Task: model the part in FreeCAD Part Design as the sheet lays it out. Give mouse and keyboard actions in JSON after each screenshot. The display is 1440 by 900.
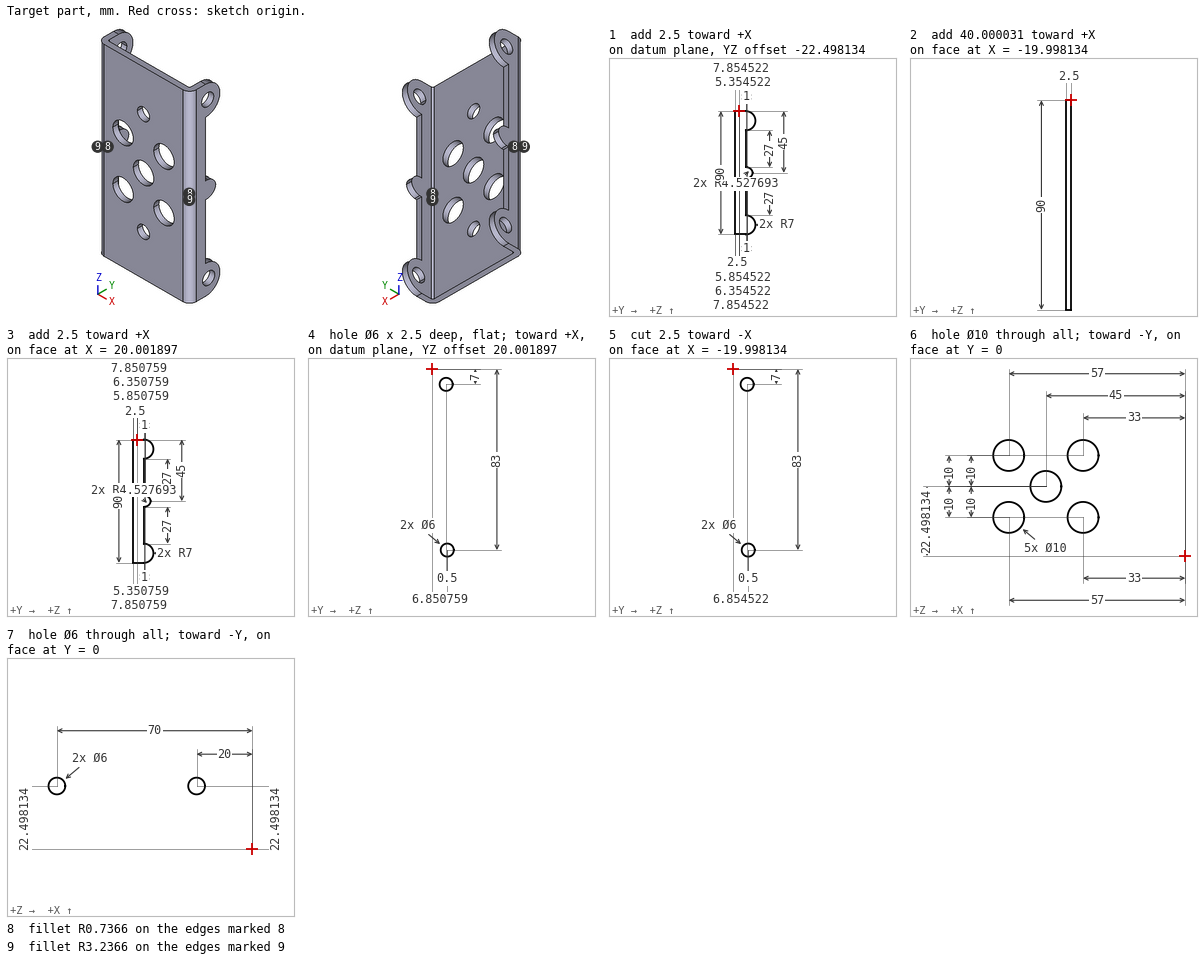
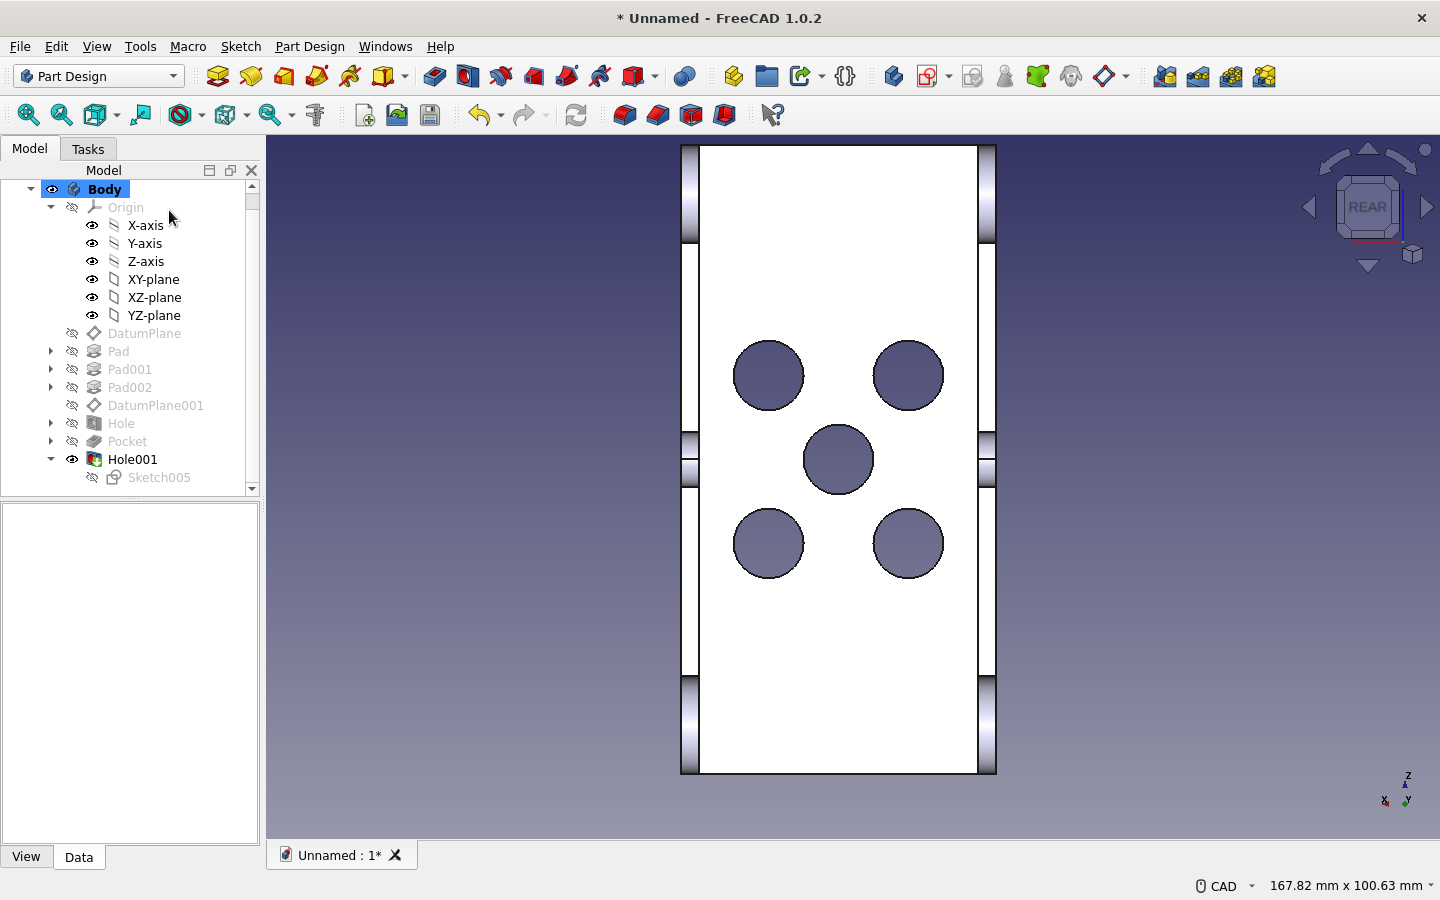
{"action": "left_click", "coordinate": [838, 279]}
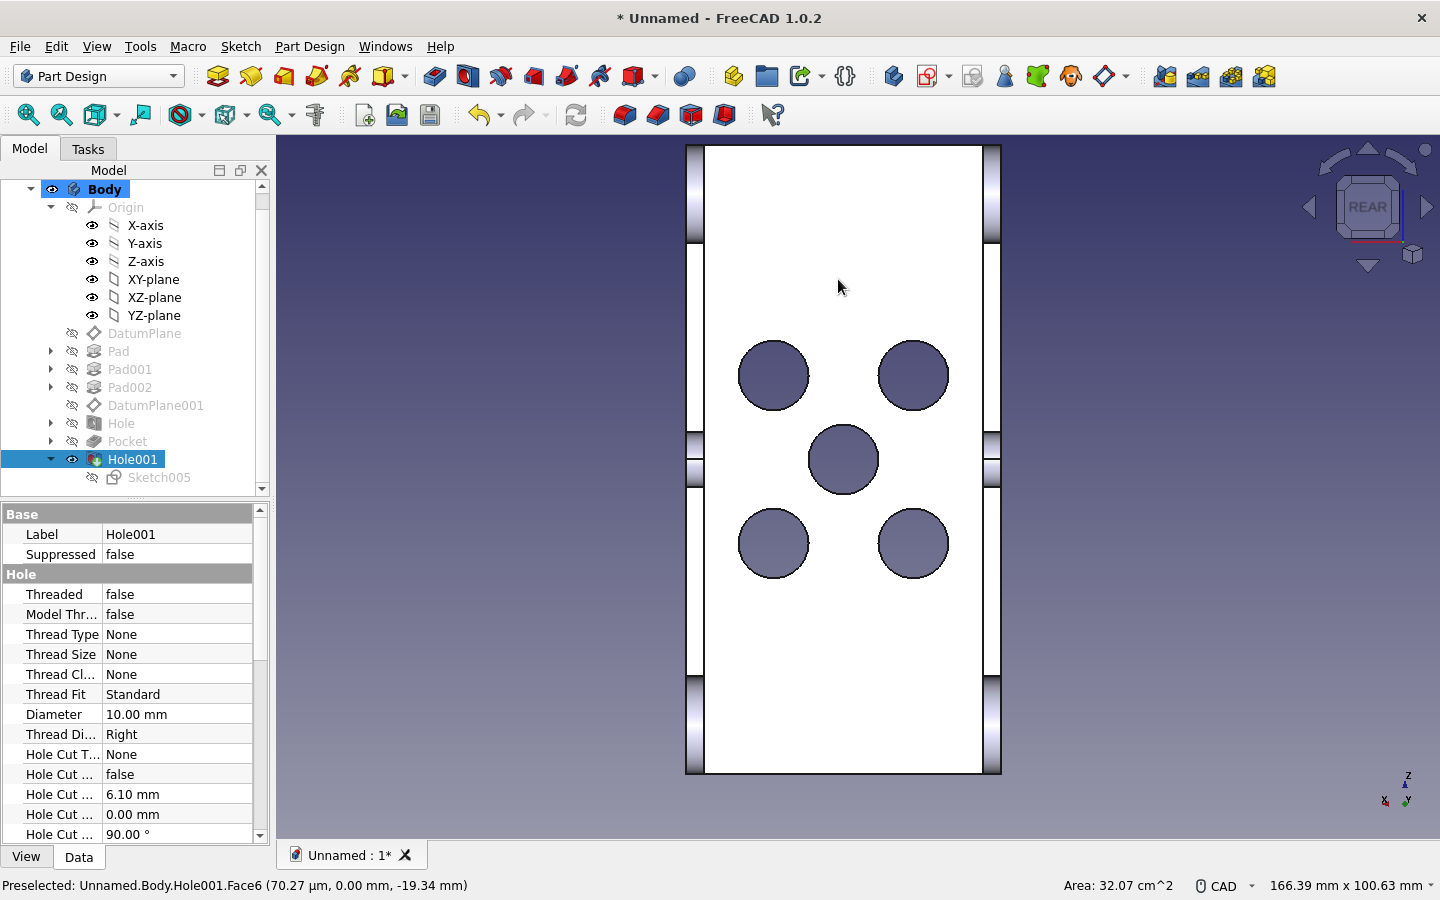
{"action": "left_click", "coordinate": [926, 76]}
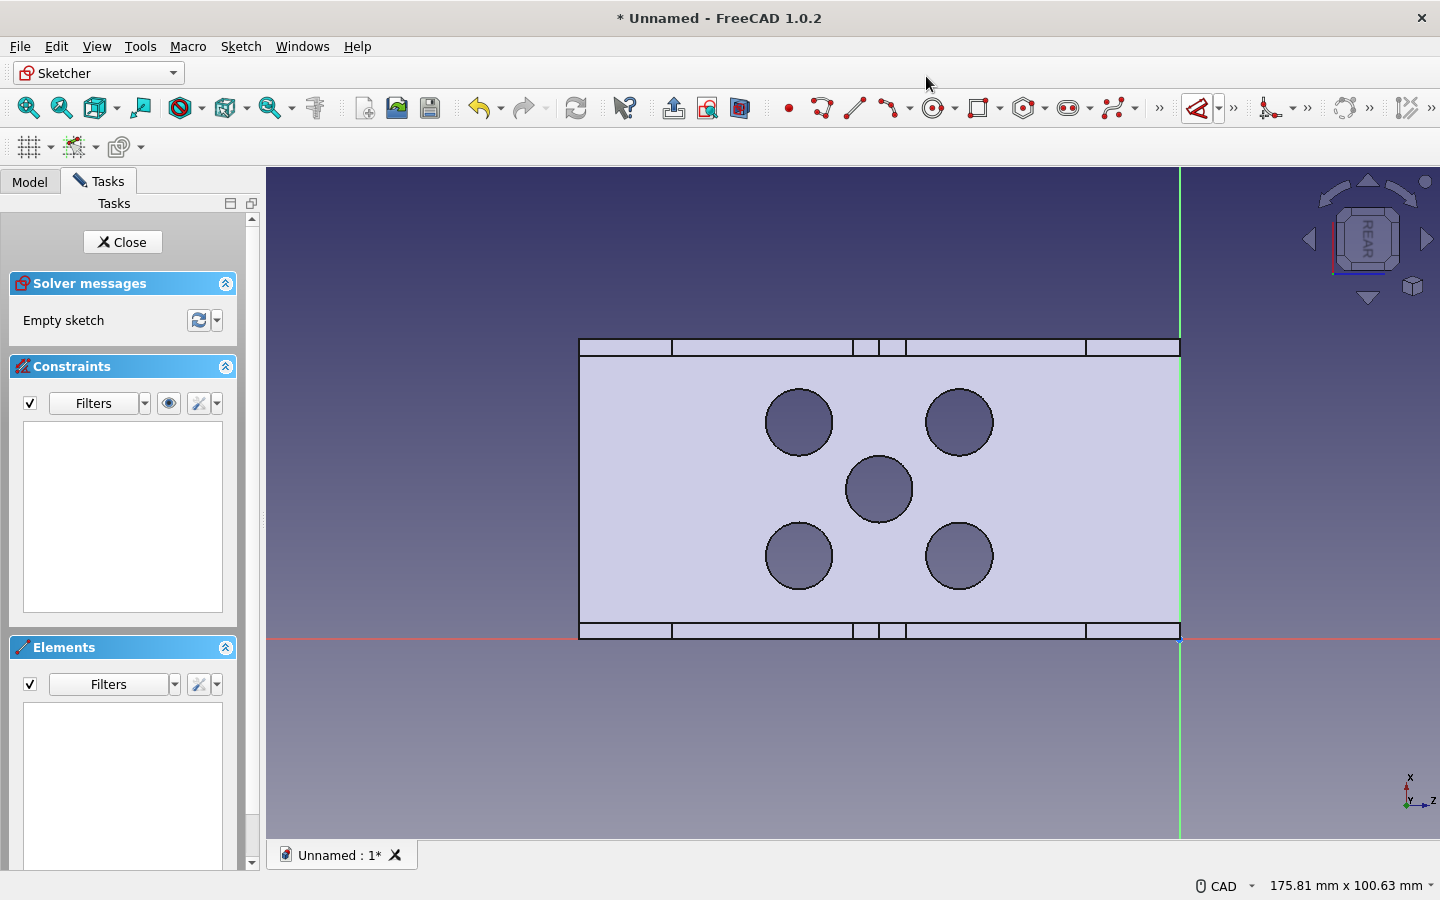
{"action": "scroll", "coordinate": [1244, 658], "scroll_direction": "up", "scroll_amount": 2}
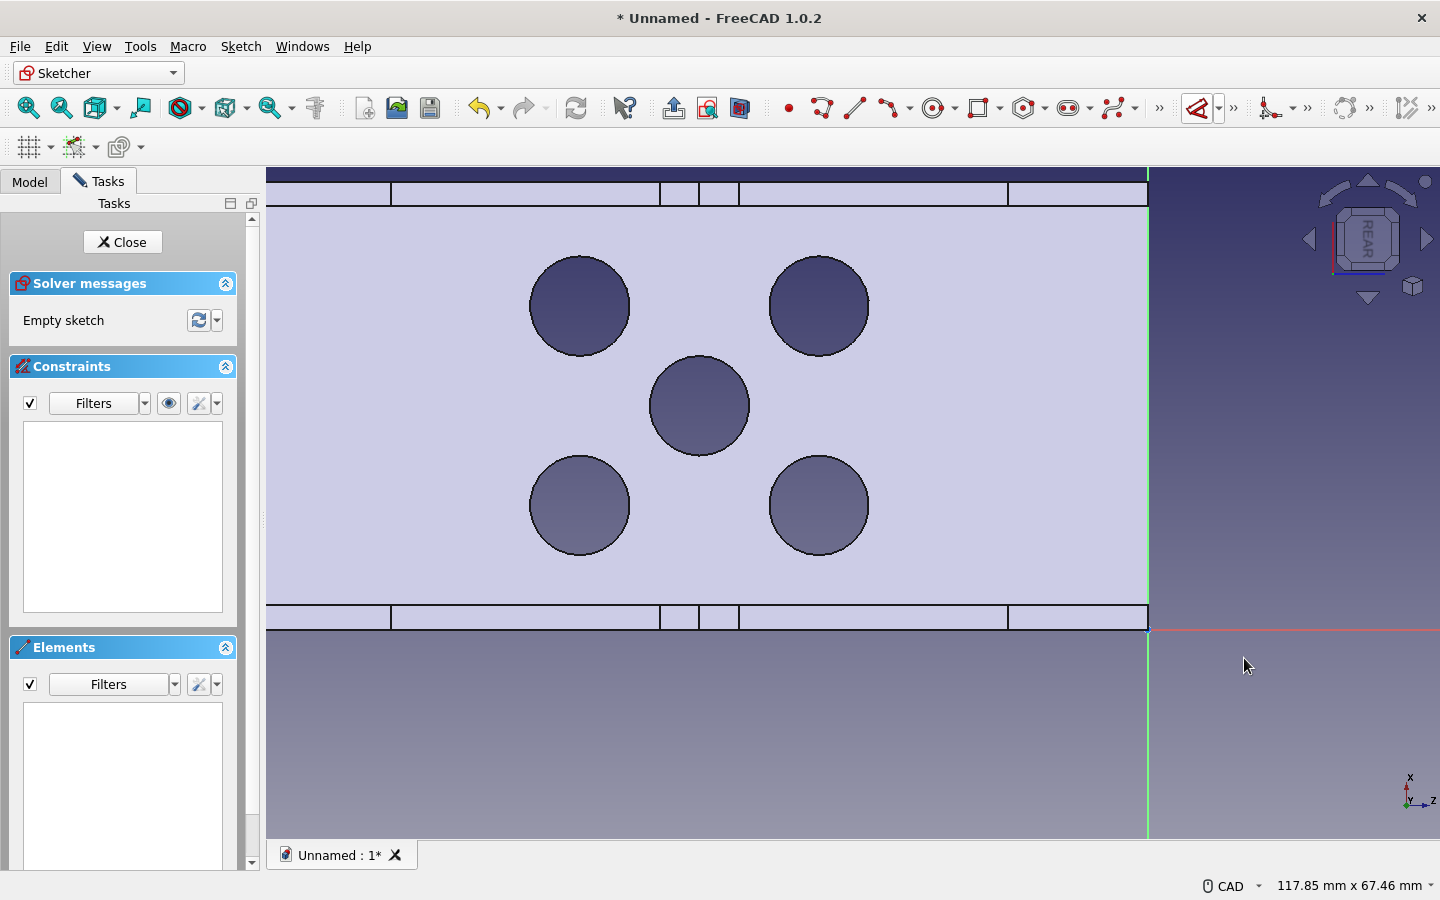
{"action": "left_click", "coordinate": [932, 108]}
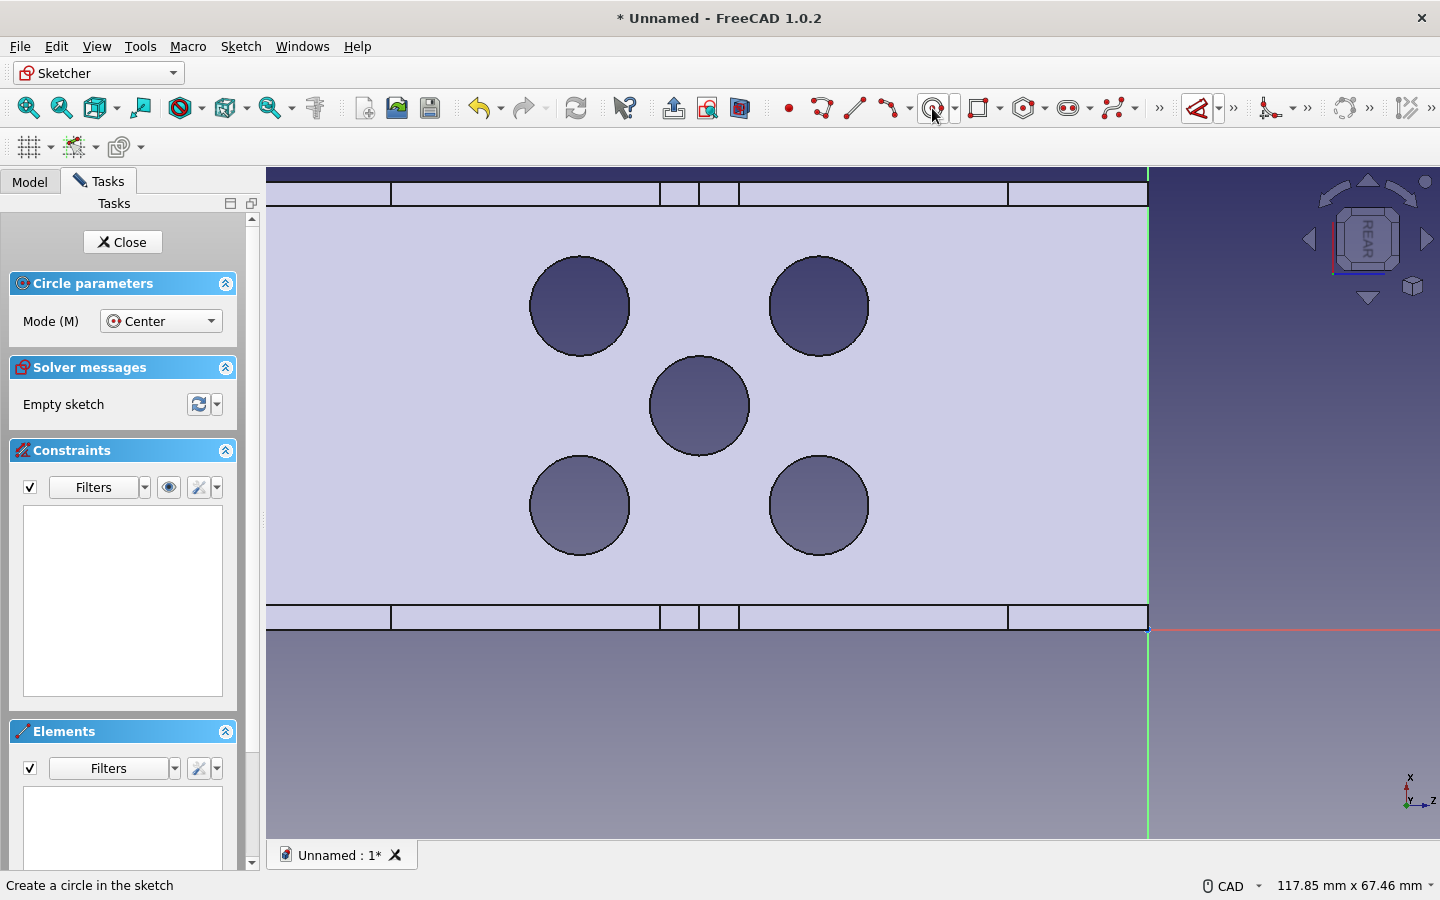
{"action": "left_click", "coordinate": [450, 406]}
{"action": "mouse_move", "coordinate": [472, 385]}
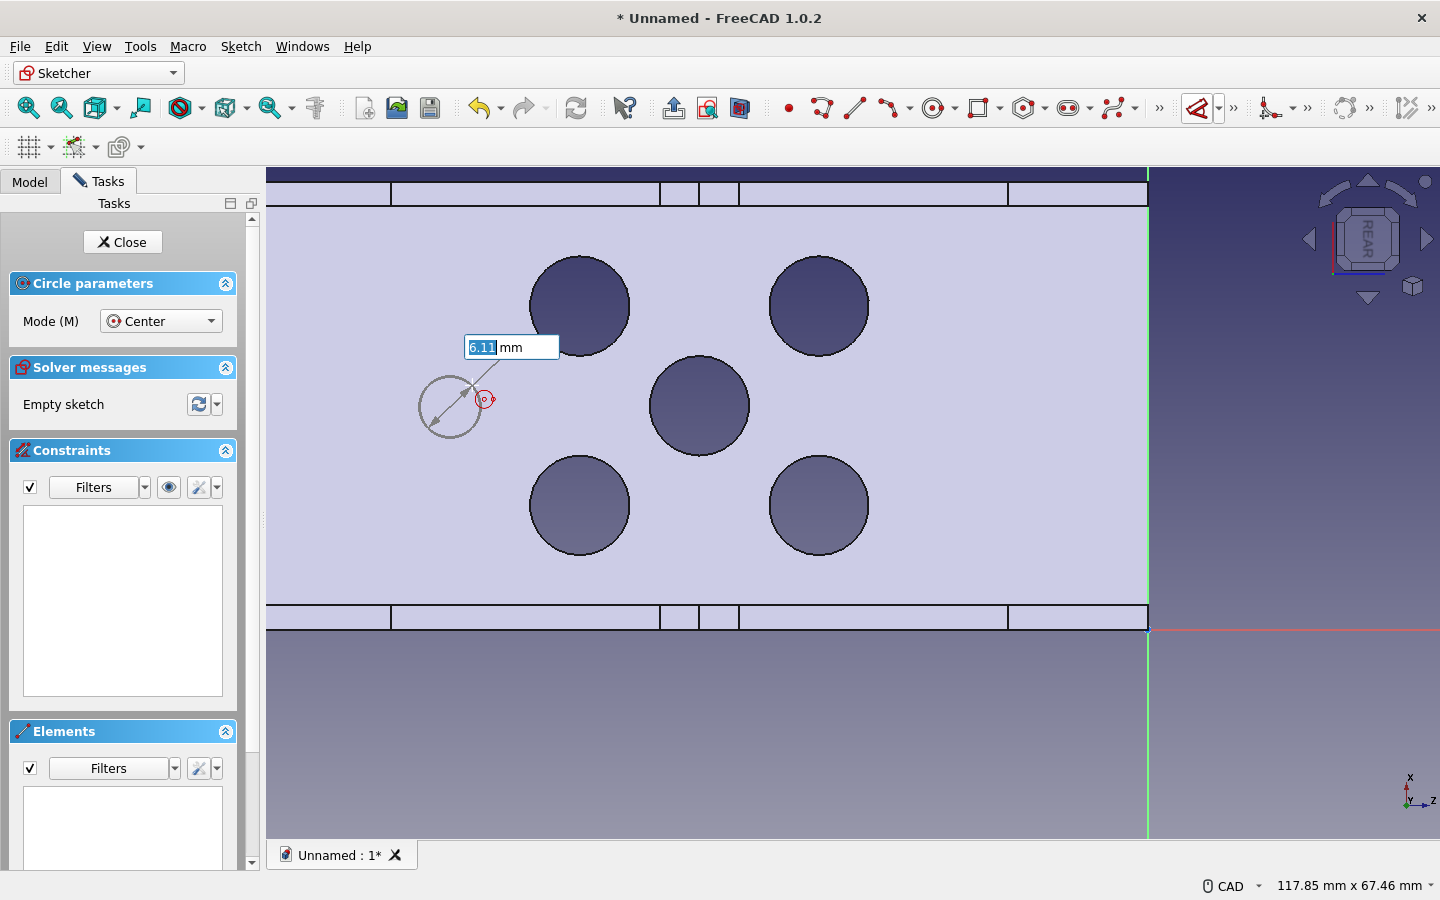
{"action": "type", "text": "6"}
{"action": "key", "text": "Return"}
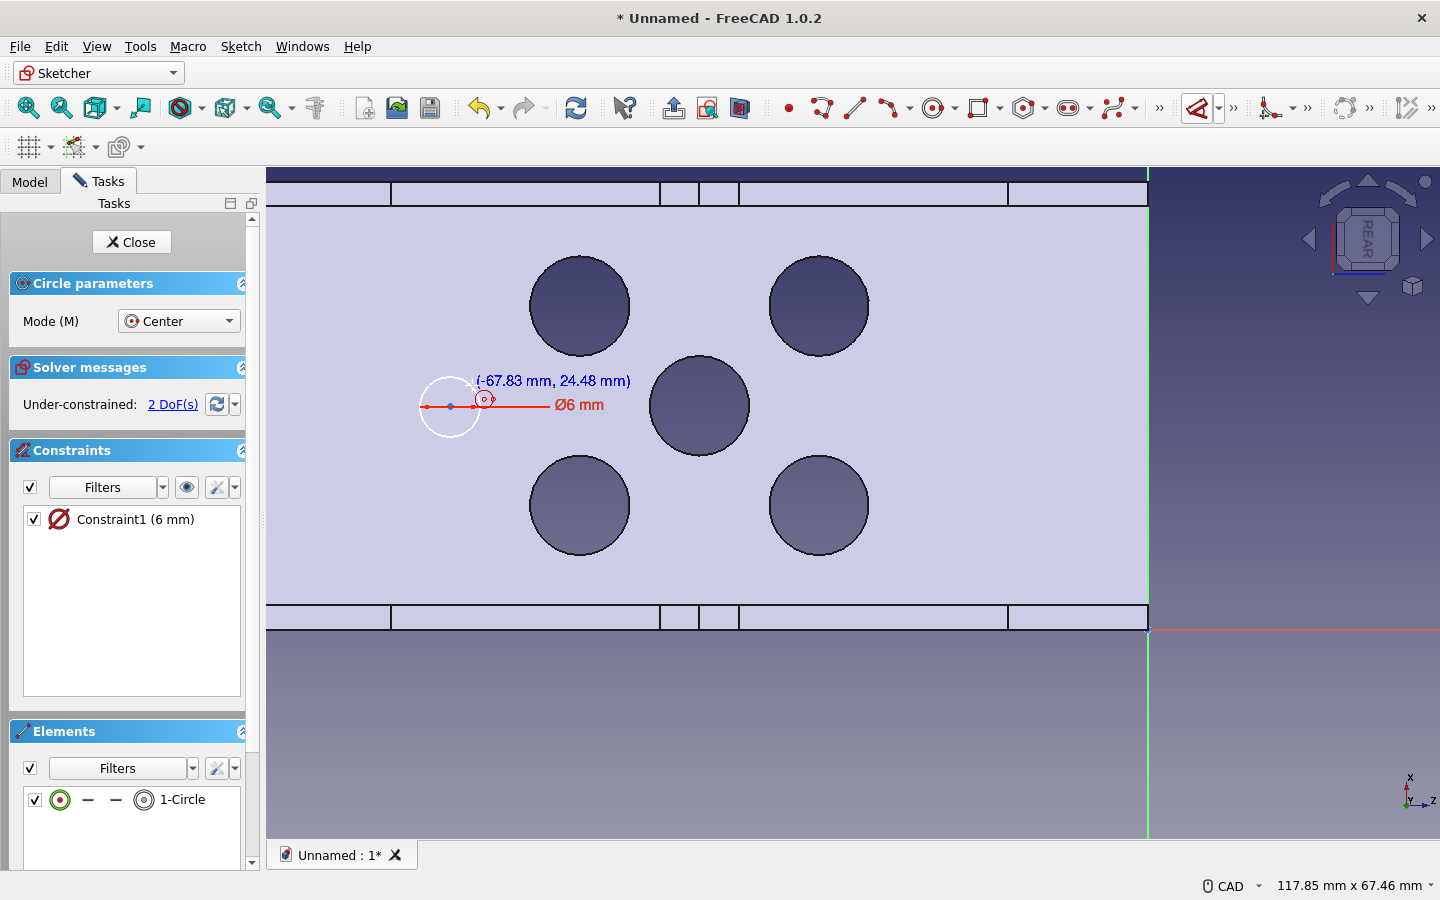
{"action": "left_click", "coordinate": [949, 406]}
{"action": "mouse_move", "coordinate": [970, 385]}